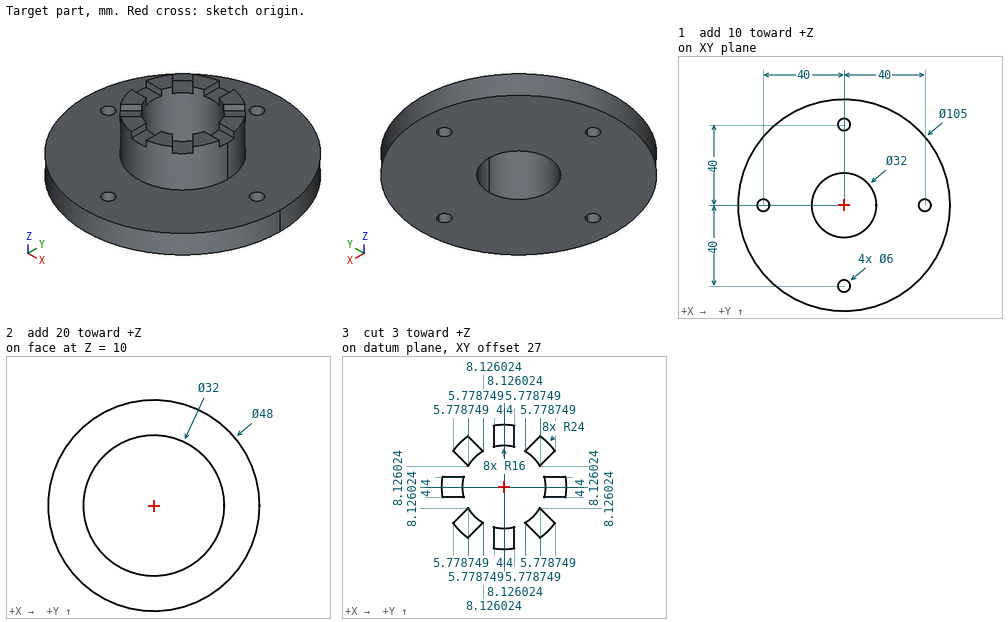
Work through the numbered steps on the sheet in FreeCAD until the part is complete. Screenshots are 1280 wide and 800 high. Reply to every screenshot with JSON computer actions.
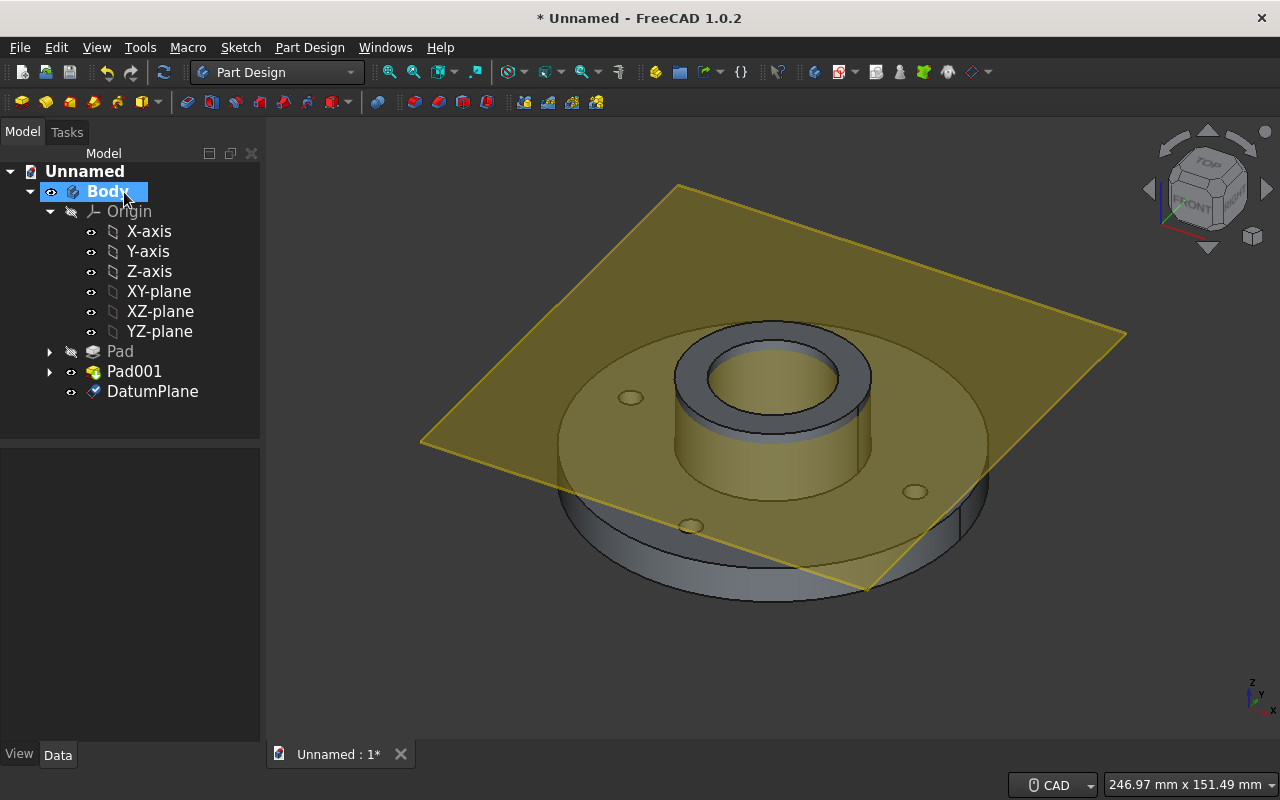
{"action": "left_click", "coordinate": [116, 392]}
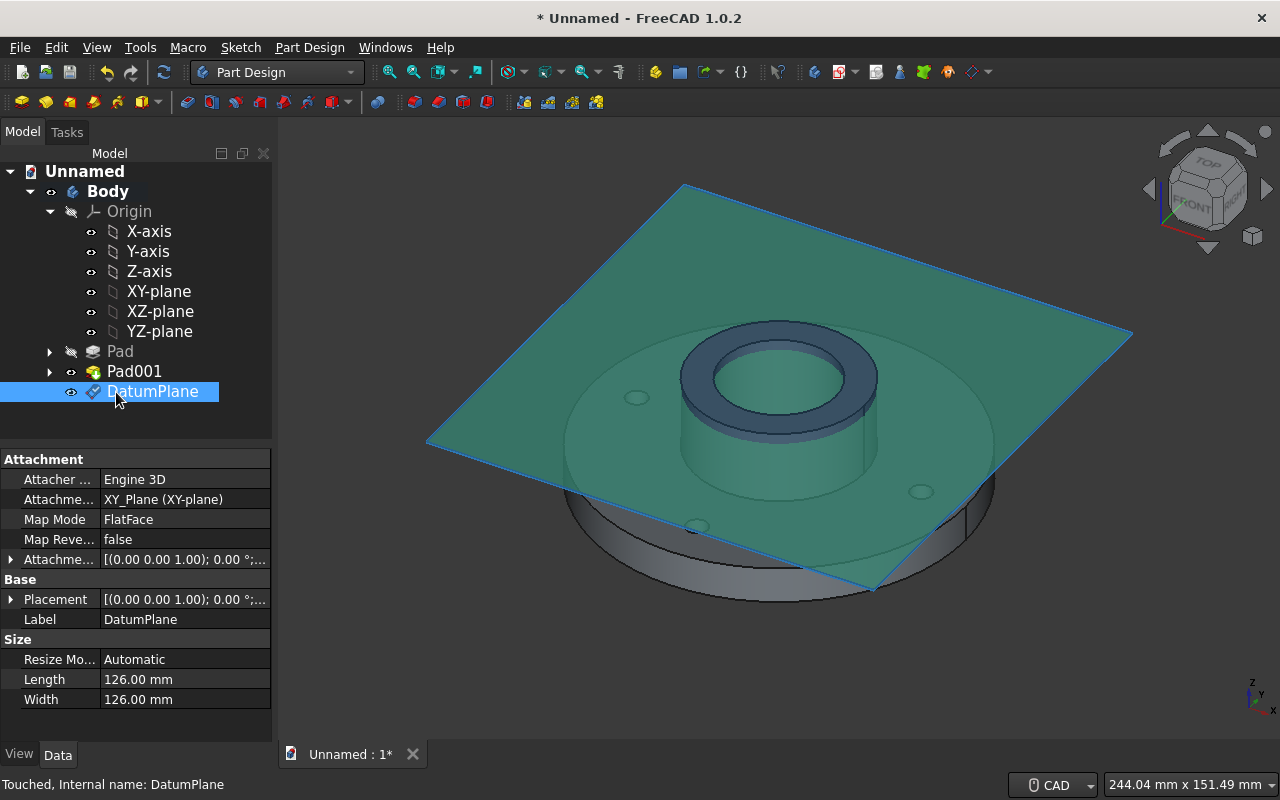
{"action": "left_click", "coordinate": [840, 72]}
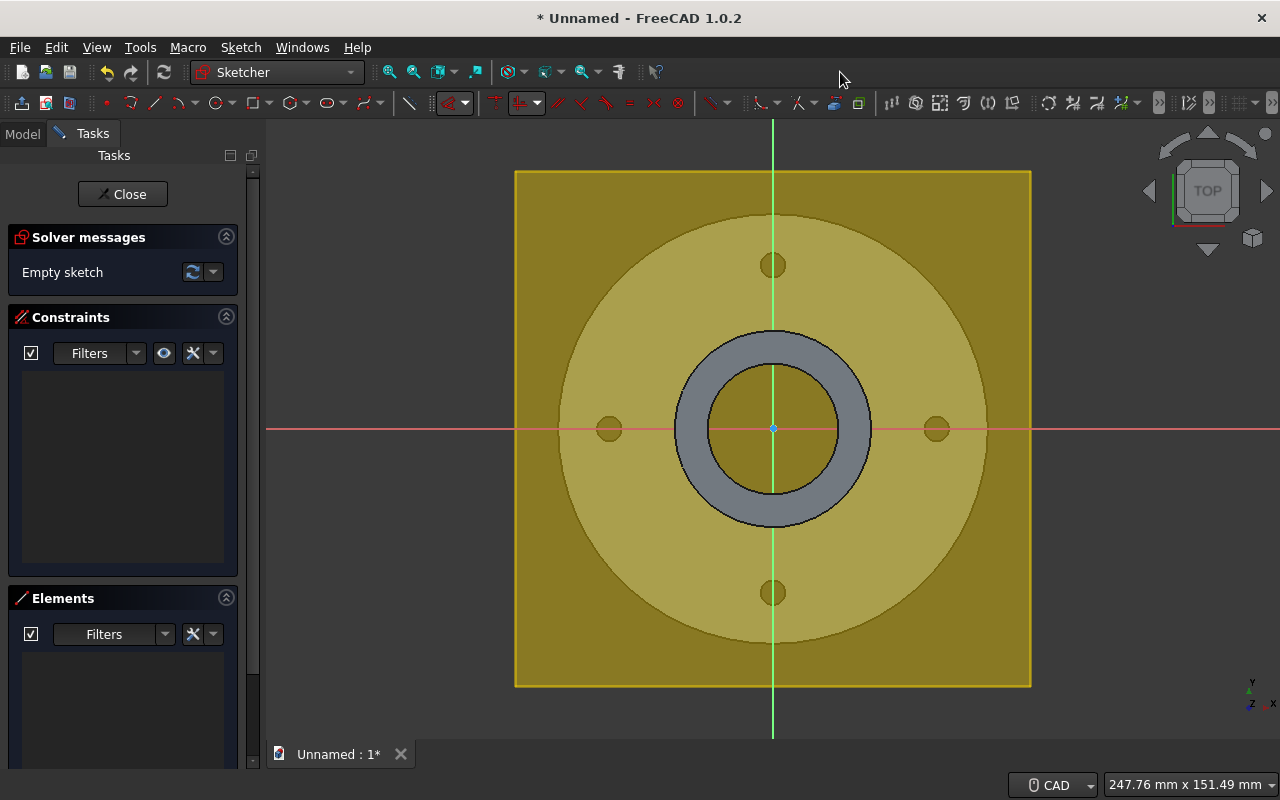
{"action": "left_click", "coordinate": [70, 104]}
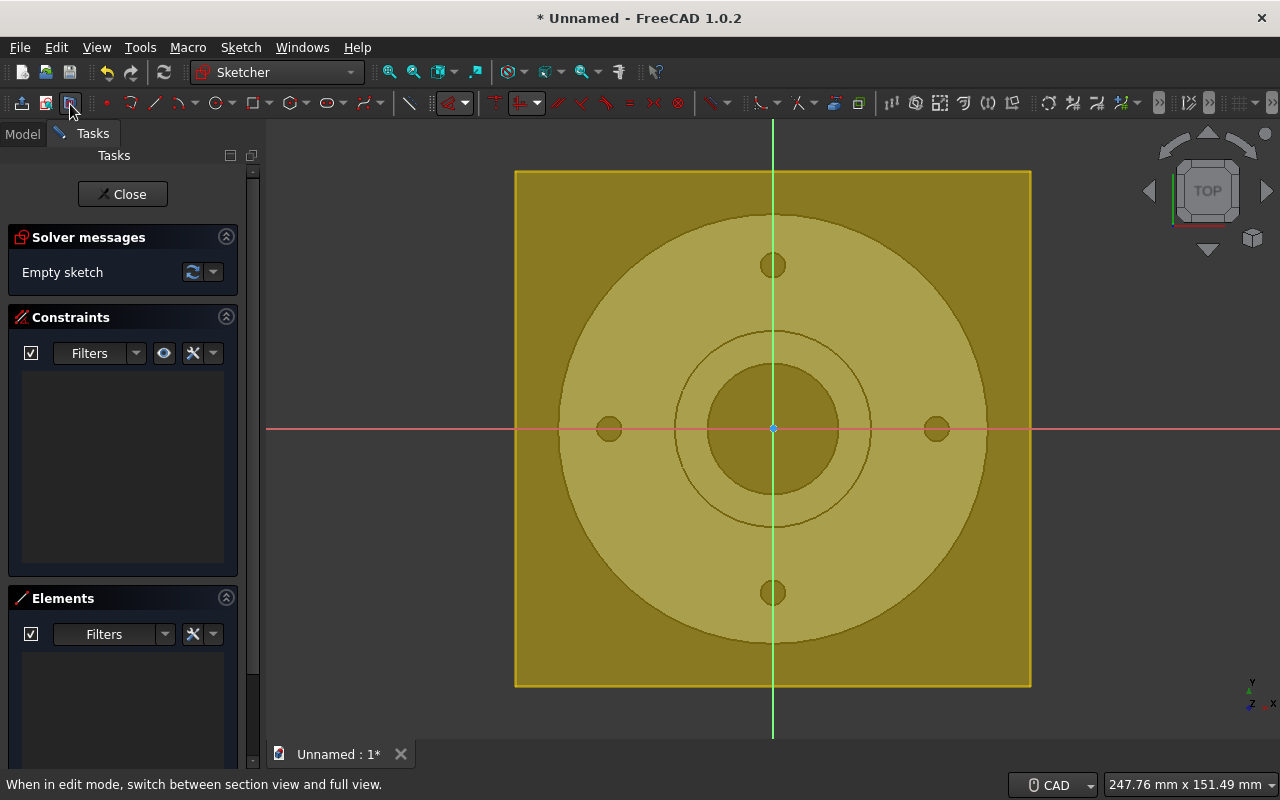
{"action": "scroll", "coordinate": [829, 429], "scroll_direction": "up", "scroll_amount": 4}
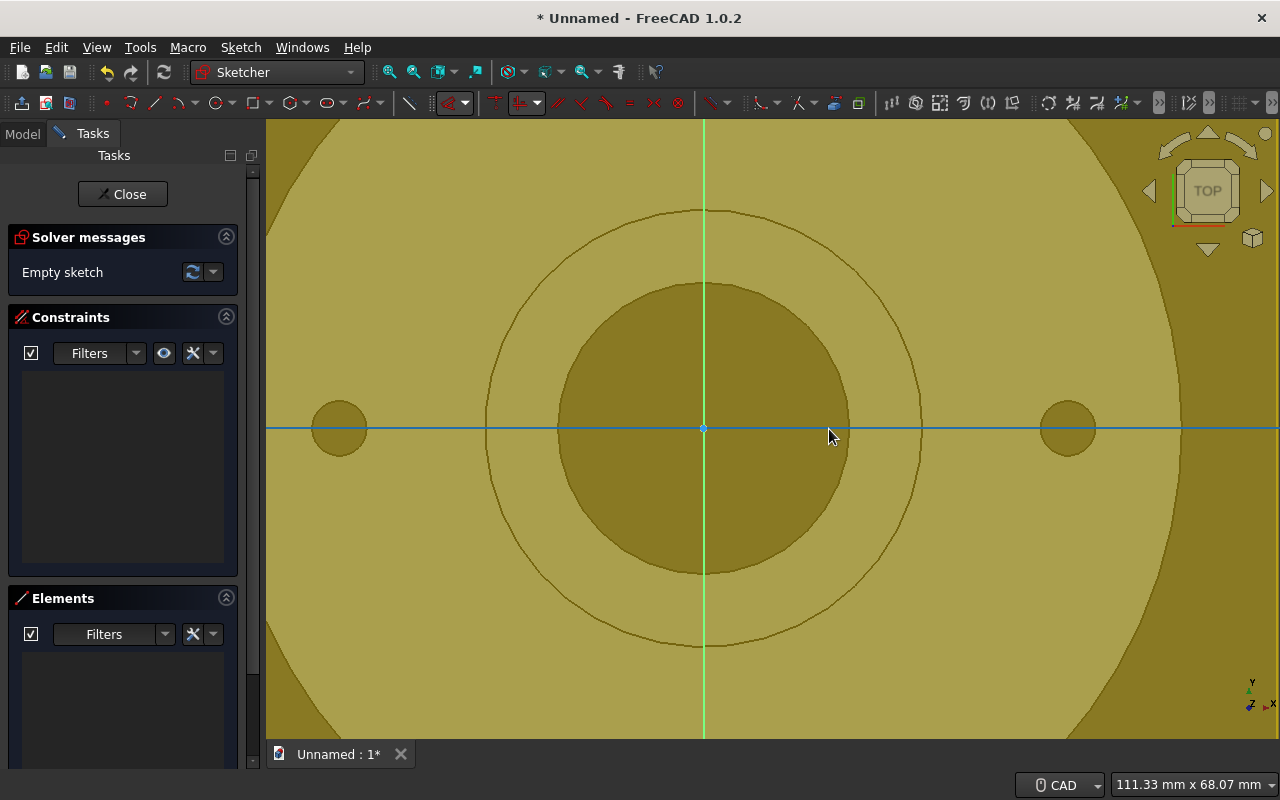
{"action": "left_click", "coordinate": [156, 104]}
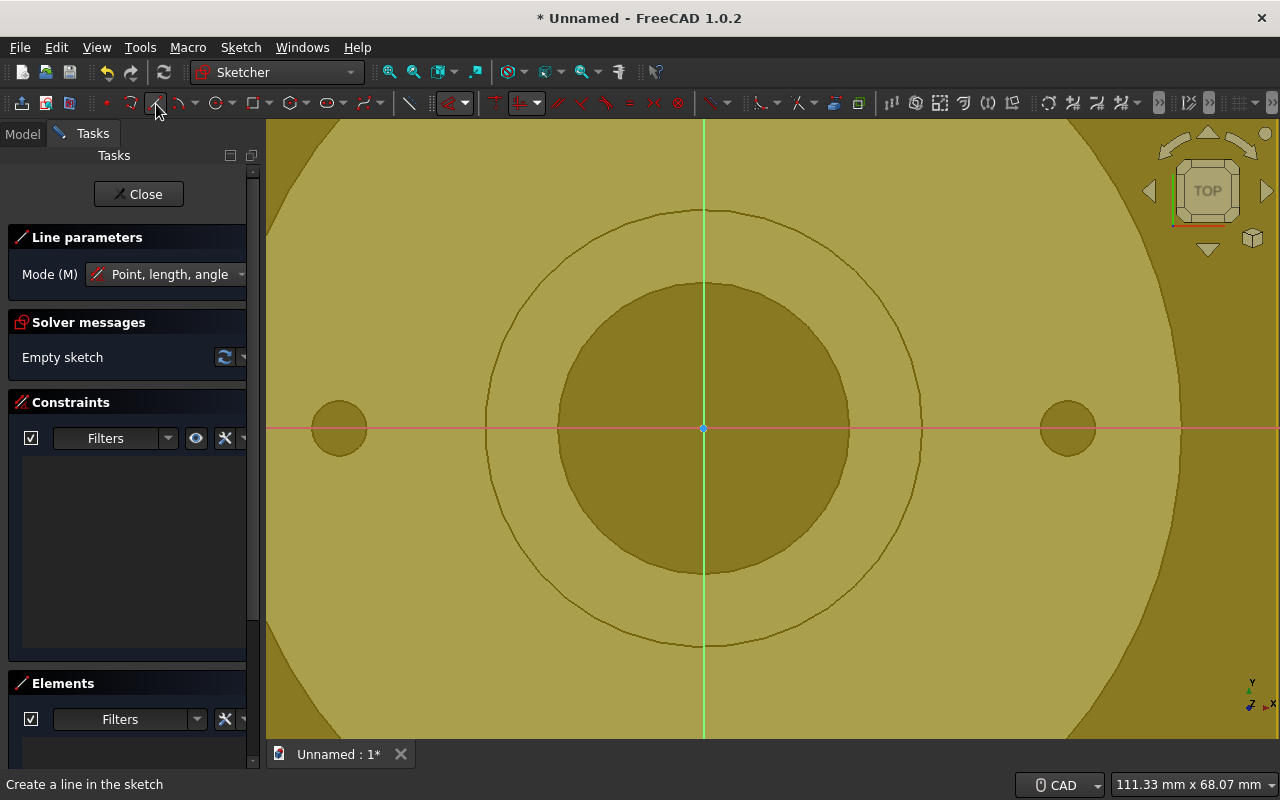
{"action": "left_click", "coordinate": [667, 213]}
{"action": "left_click", "coordinate": [667, 287]}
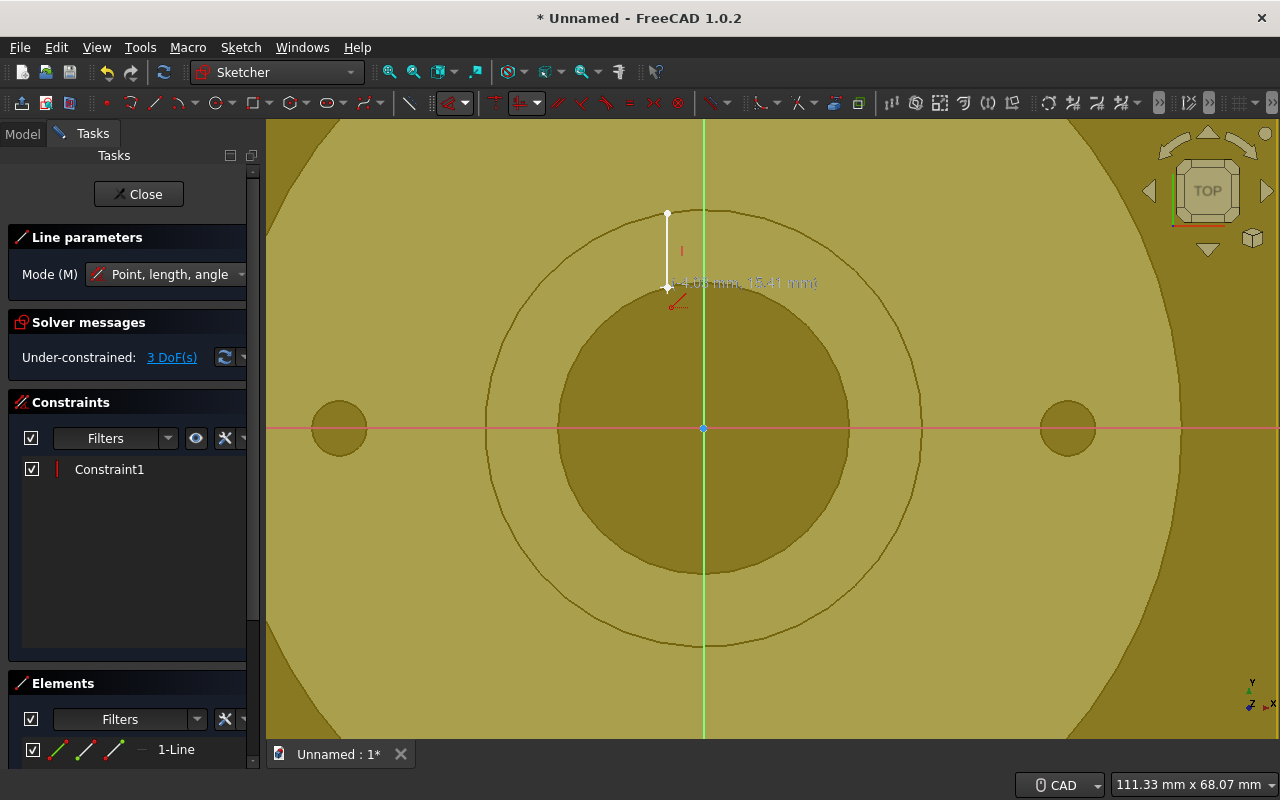
{"action": "left_click", "coordinate": [740, 287]}
{"action": "left_click", "coordinate": [740, 213]}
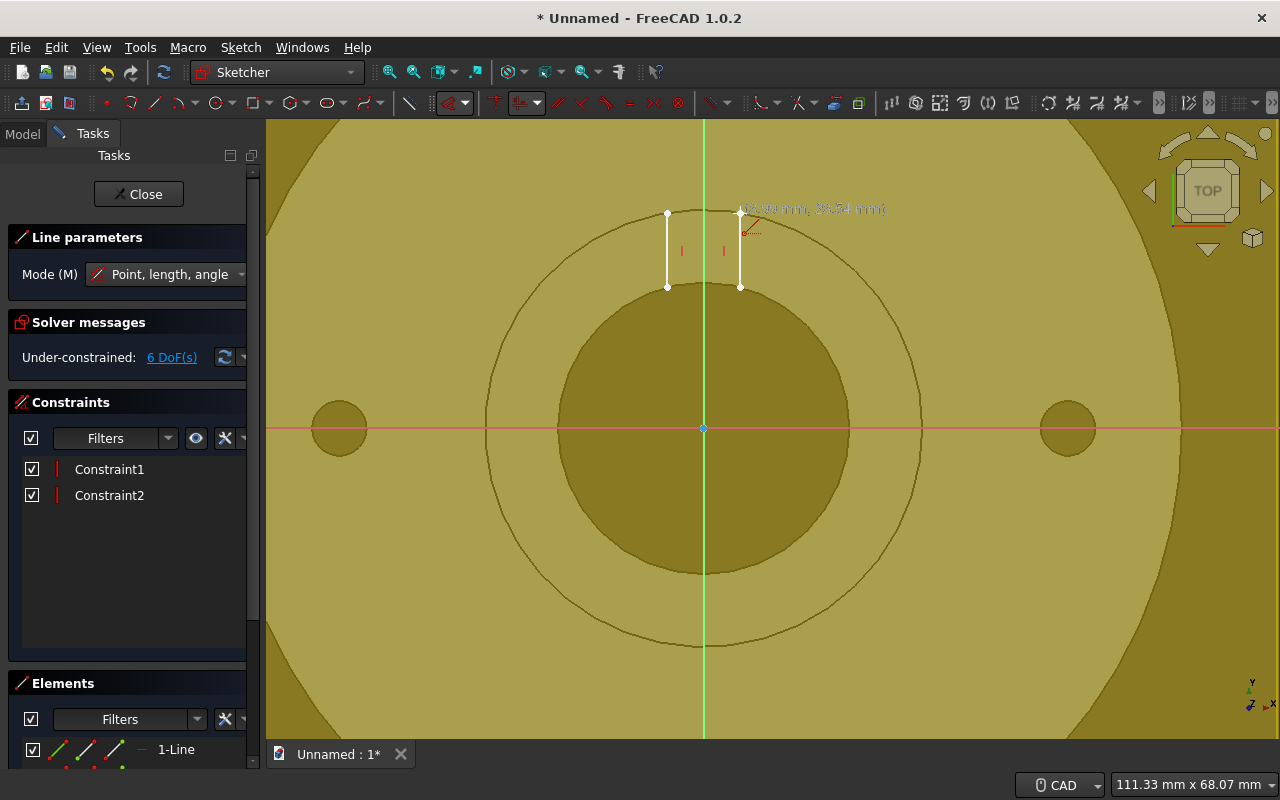
{"action": "key", "text": "g 3 a"}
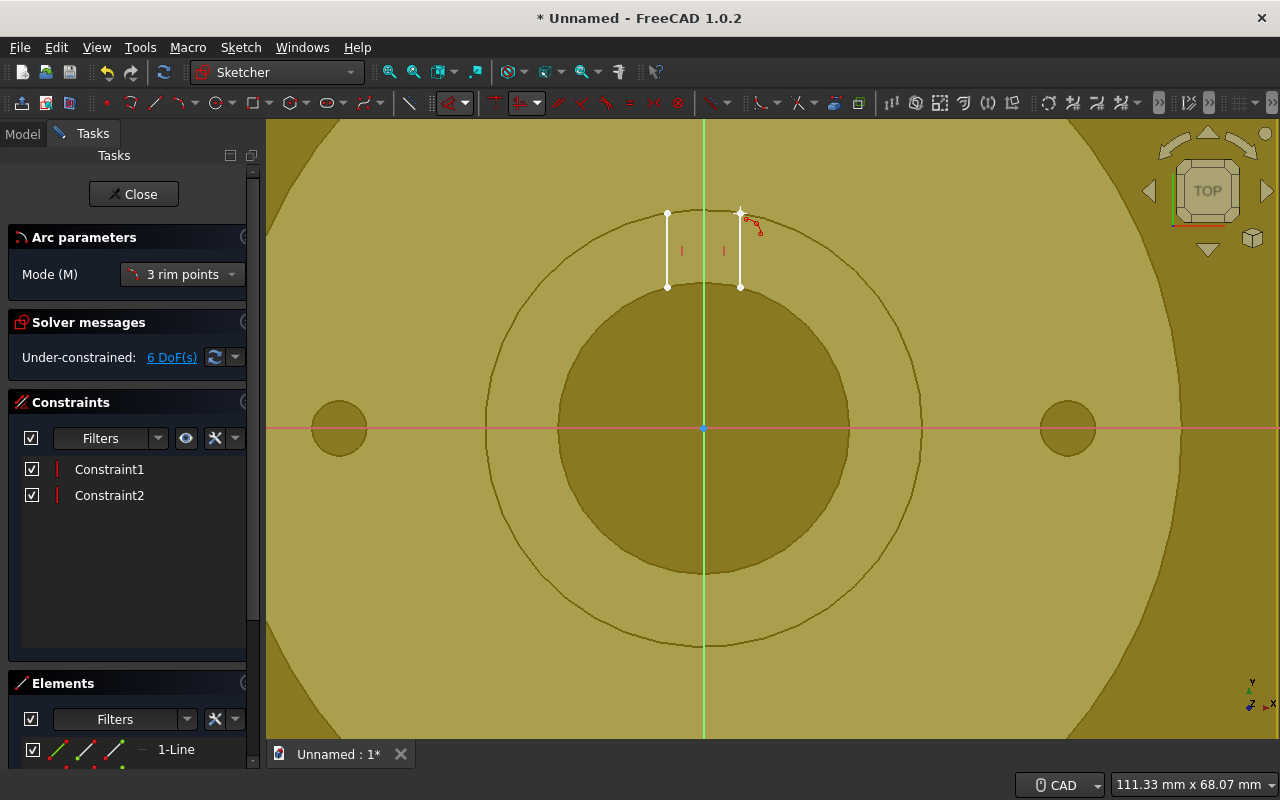
{"action": "left_click", "coordinate": [667, 288]}
{"action": "left_click", "coordinate": [740, 288]}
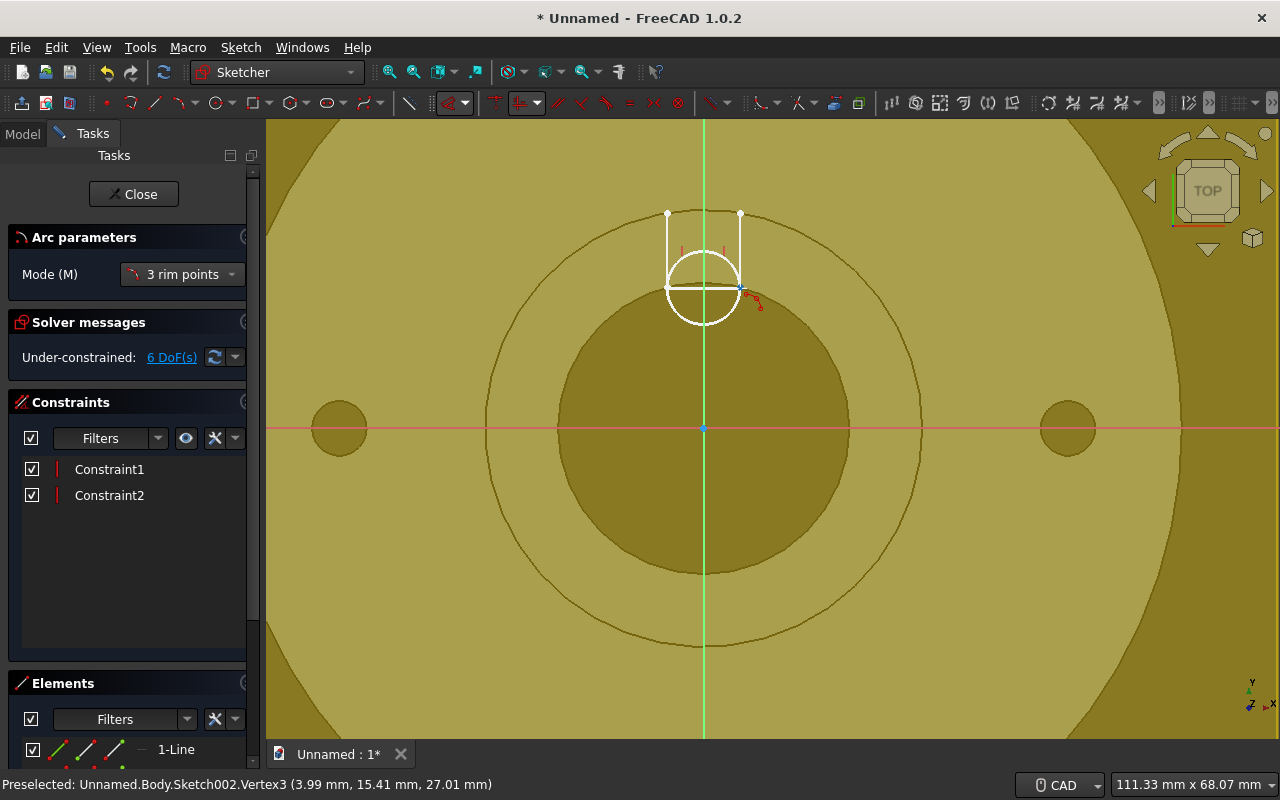
{"action": "scroll", "coordinate": [711, 283], "scroll_direction": "up", "scroll_amount": 7}